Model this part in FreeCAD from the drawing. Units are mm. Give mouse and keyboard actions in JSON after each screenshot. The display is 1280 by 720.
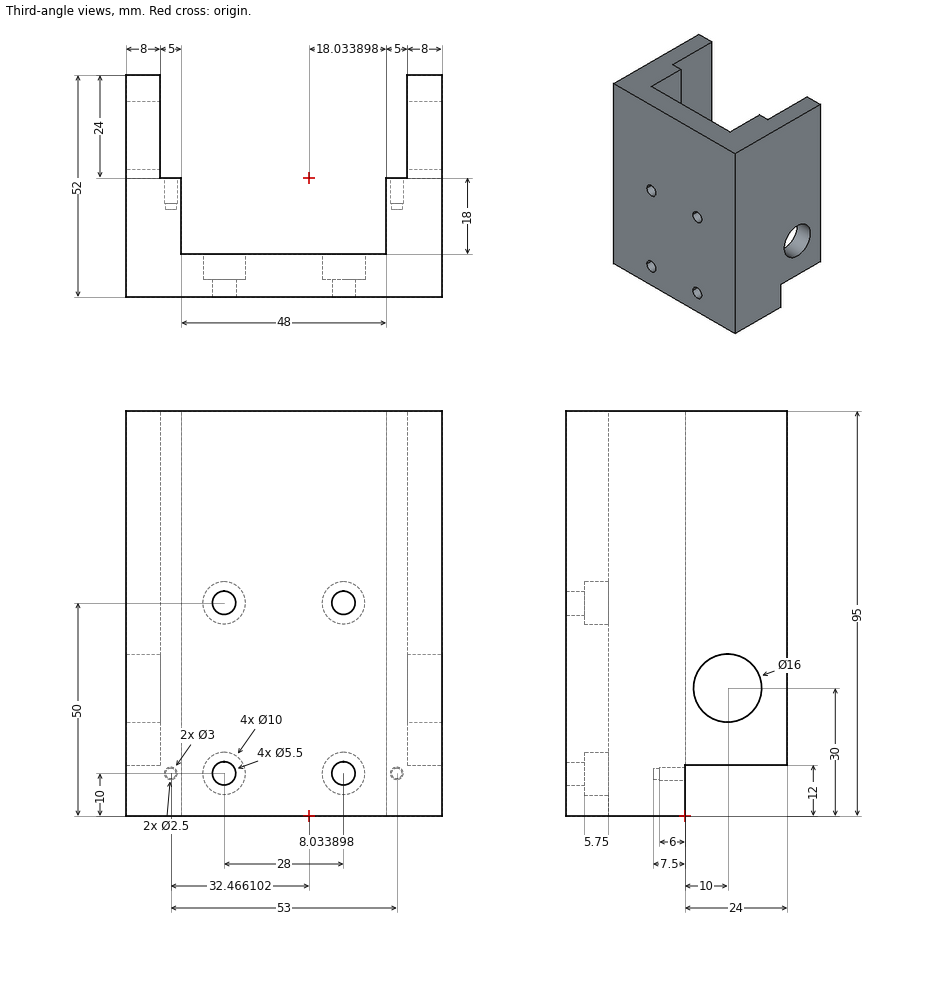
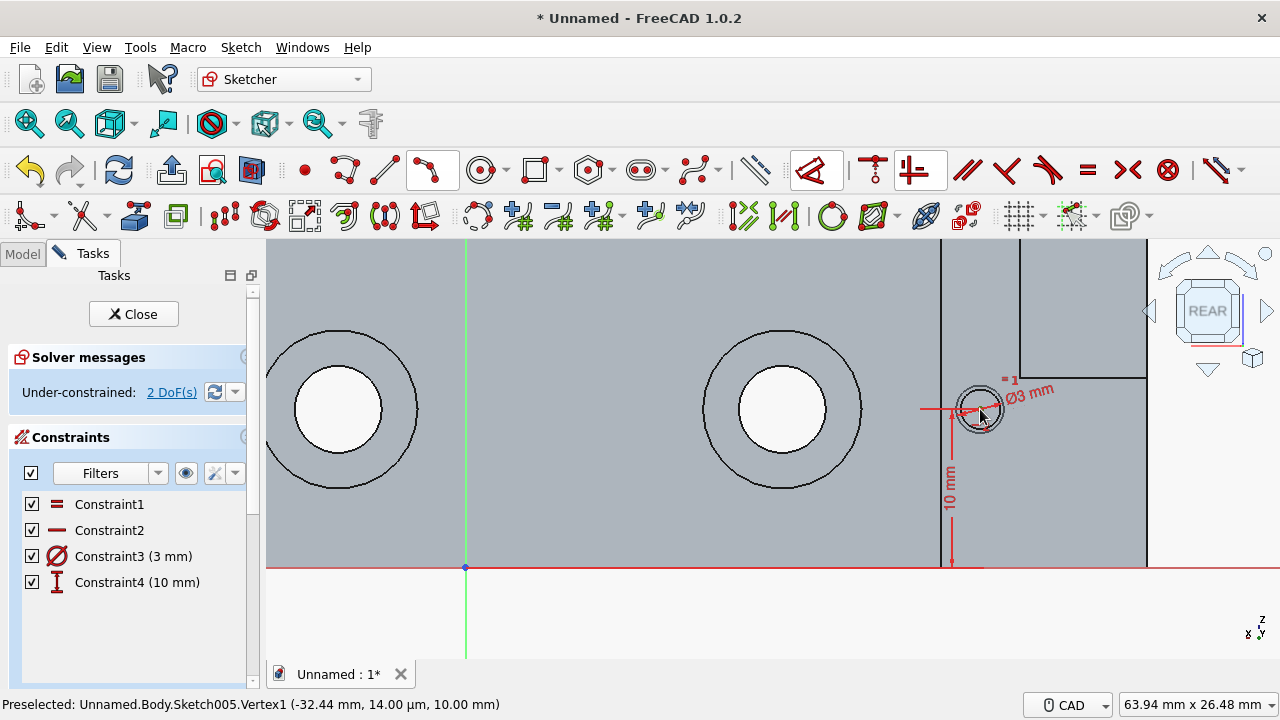
{"action": "scroll", "coordinate": [998, 393], "scroll_direction": "down", "scroll_amount": 2}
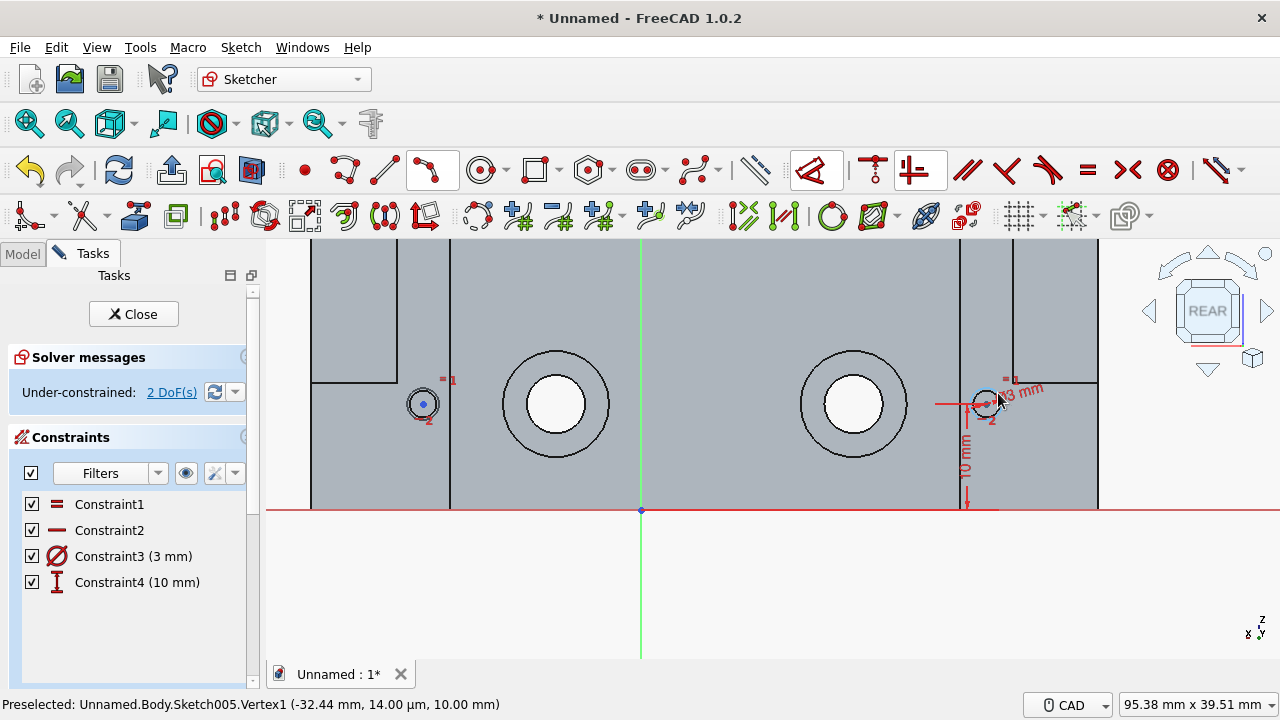
{"action": "left_click", "coordinate": [423, 404]}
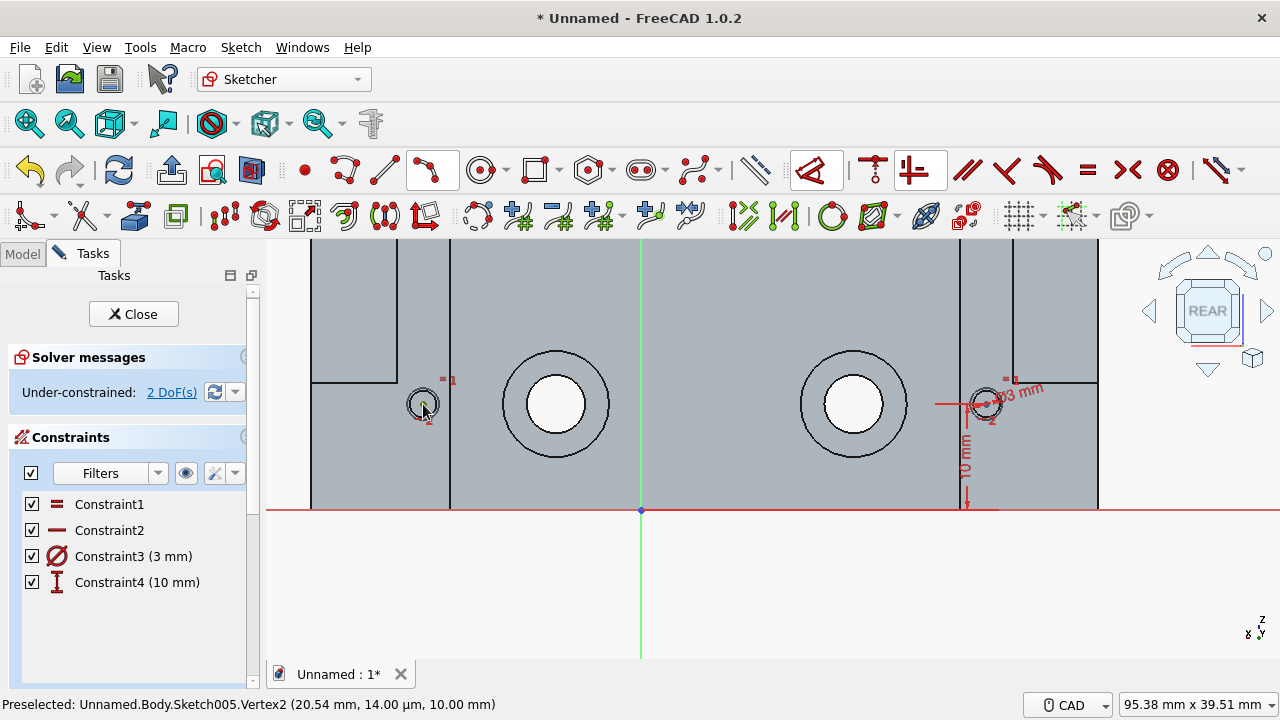
{"action": "key", "text": "l"}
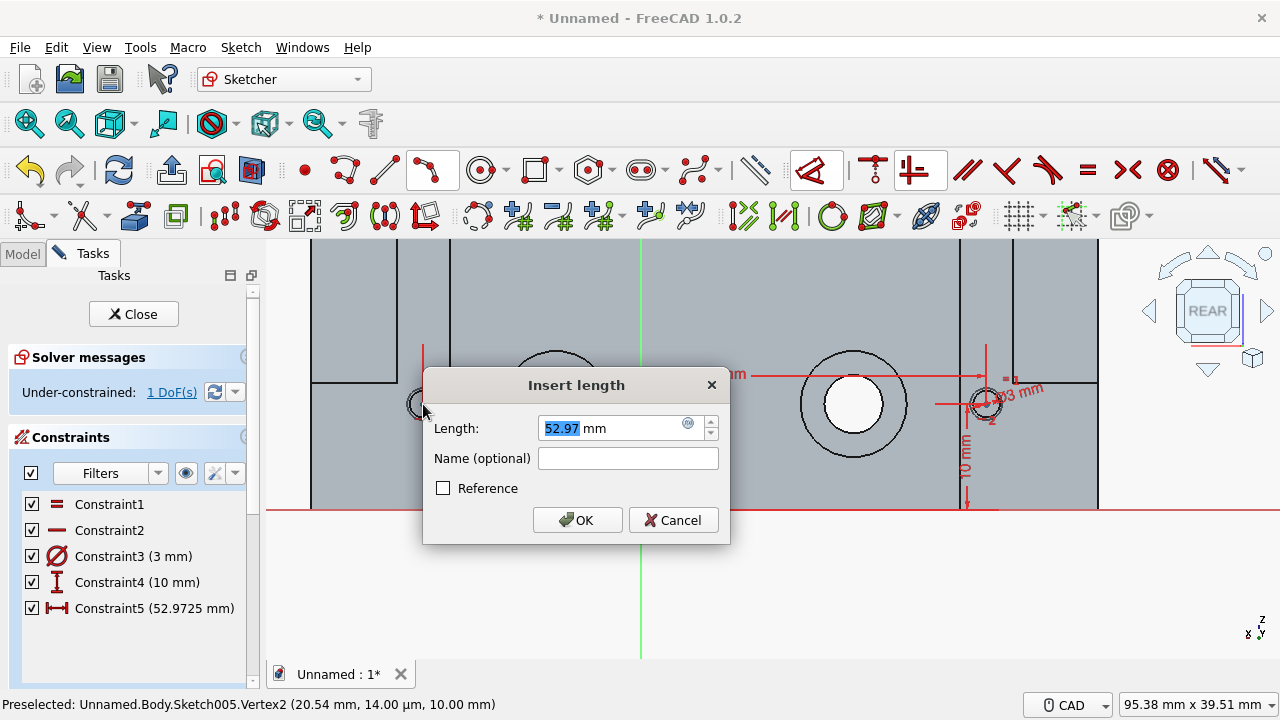
{"action": "type", "text": "53"}
{"action": "key", "text": "Return"}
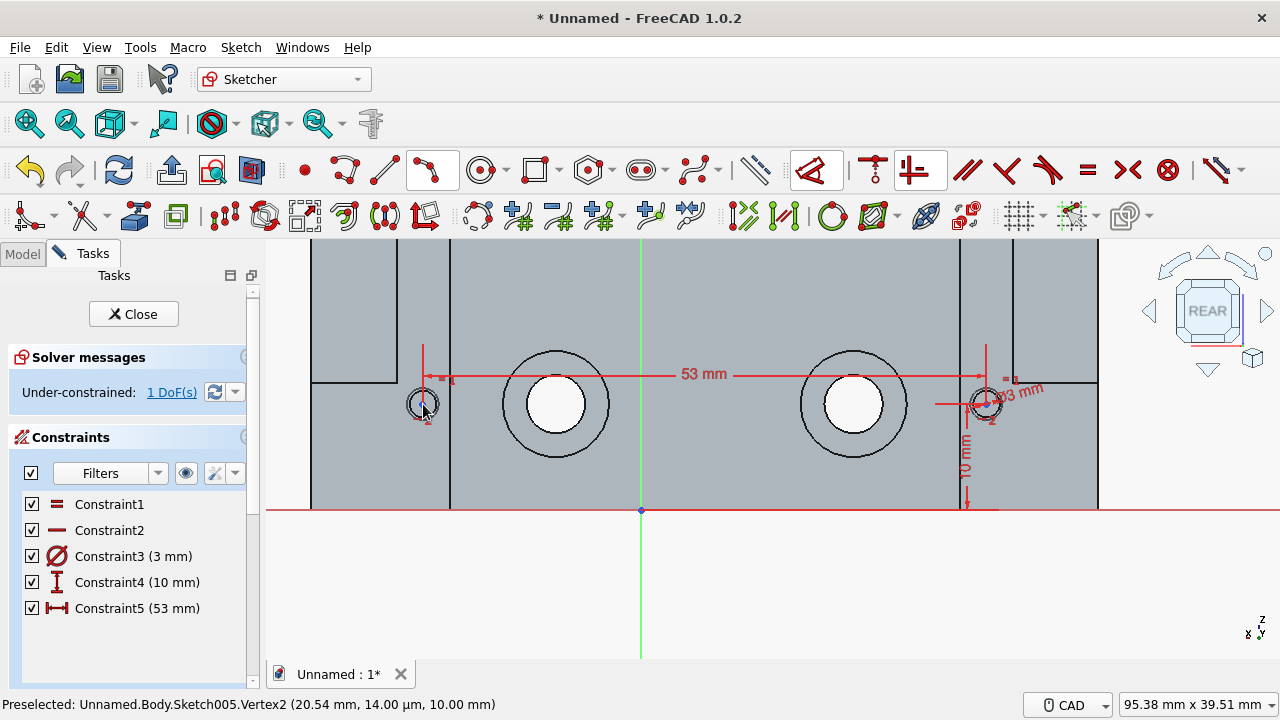
{"action": "left_click", "coordinate": [986, 404]}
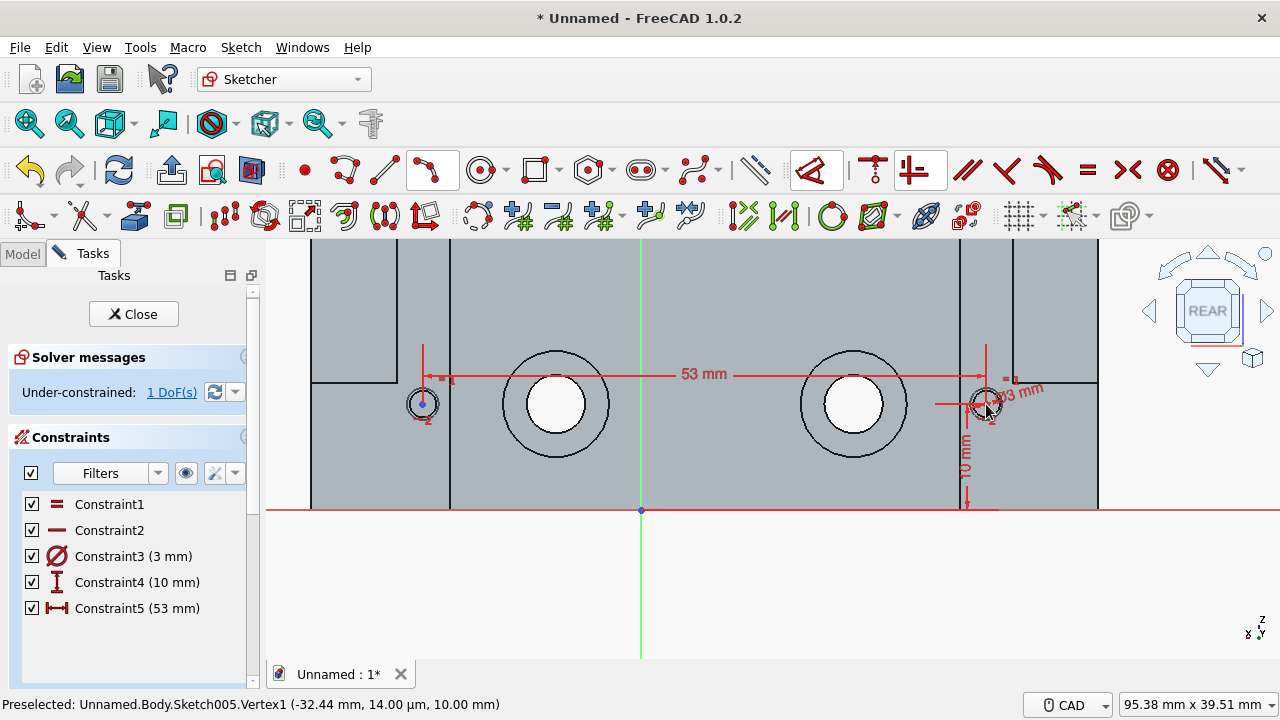
{"action": "key", "text": "l"}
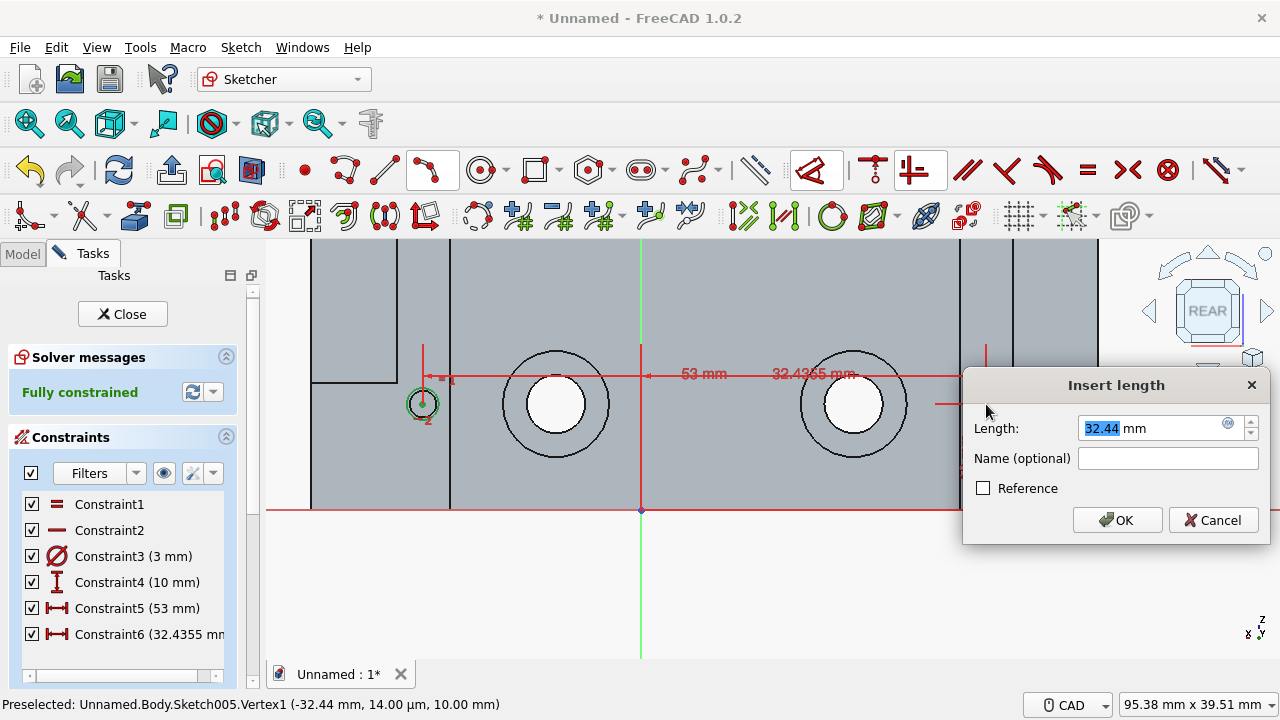
{"action": "type", "text": "32.466102"}
{"action": "key", "text": "Return"}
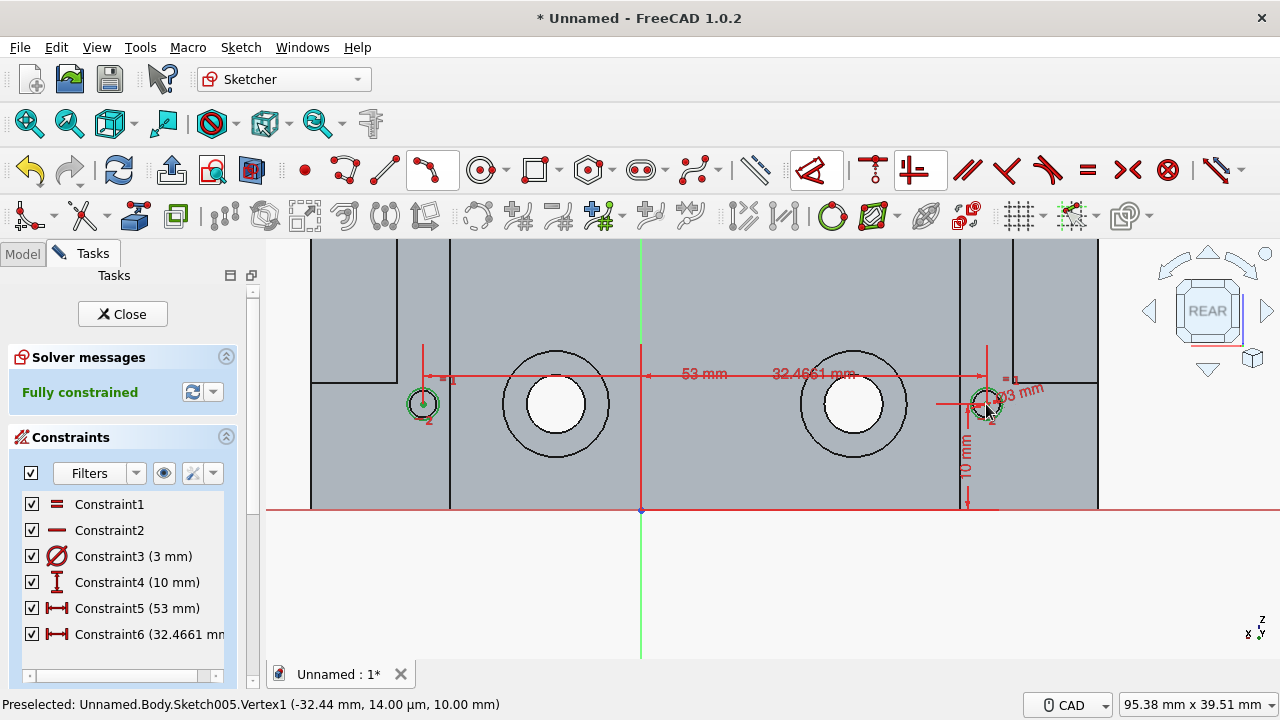
{"action": "left_click", "coordinate": [123, 314]}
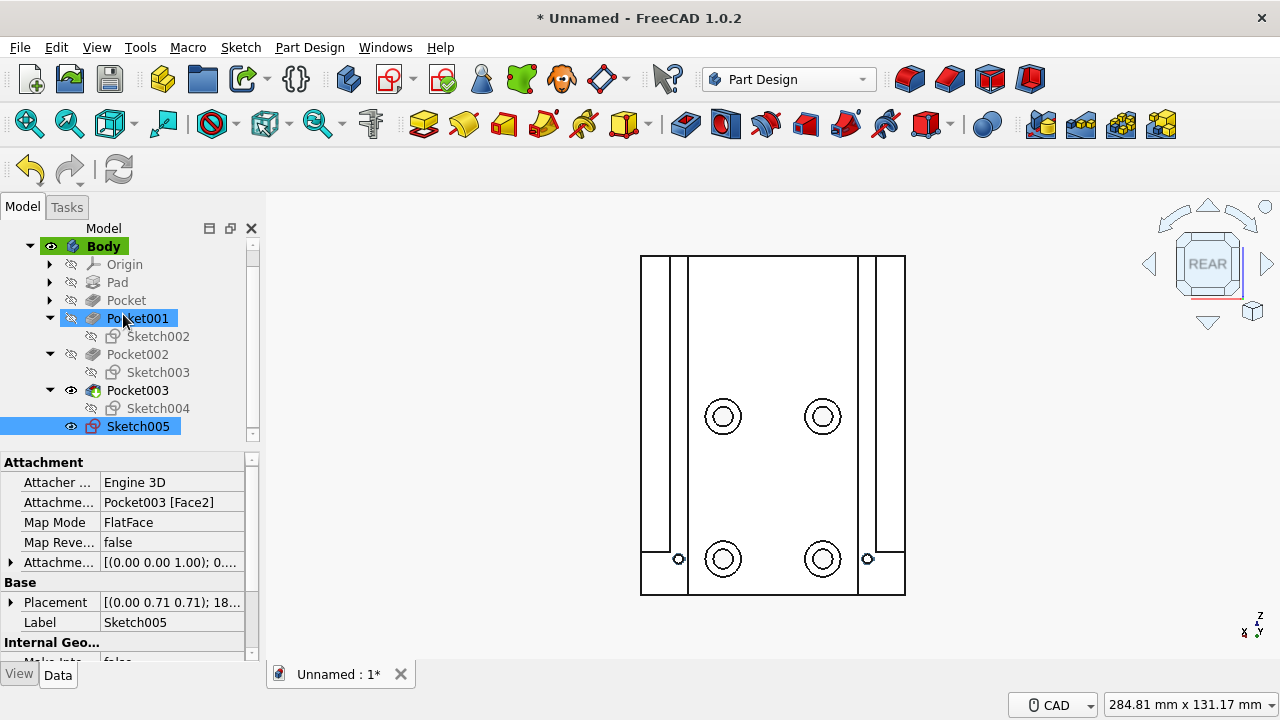
{"action": "left_click", "coordinate": [686, 124]}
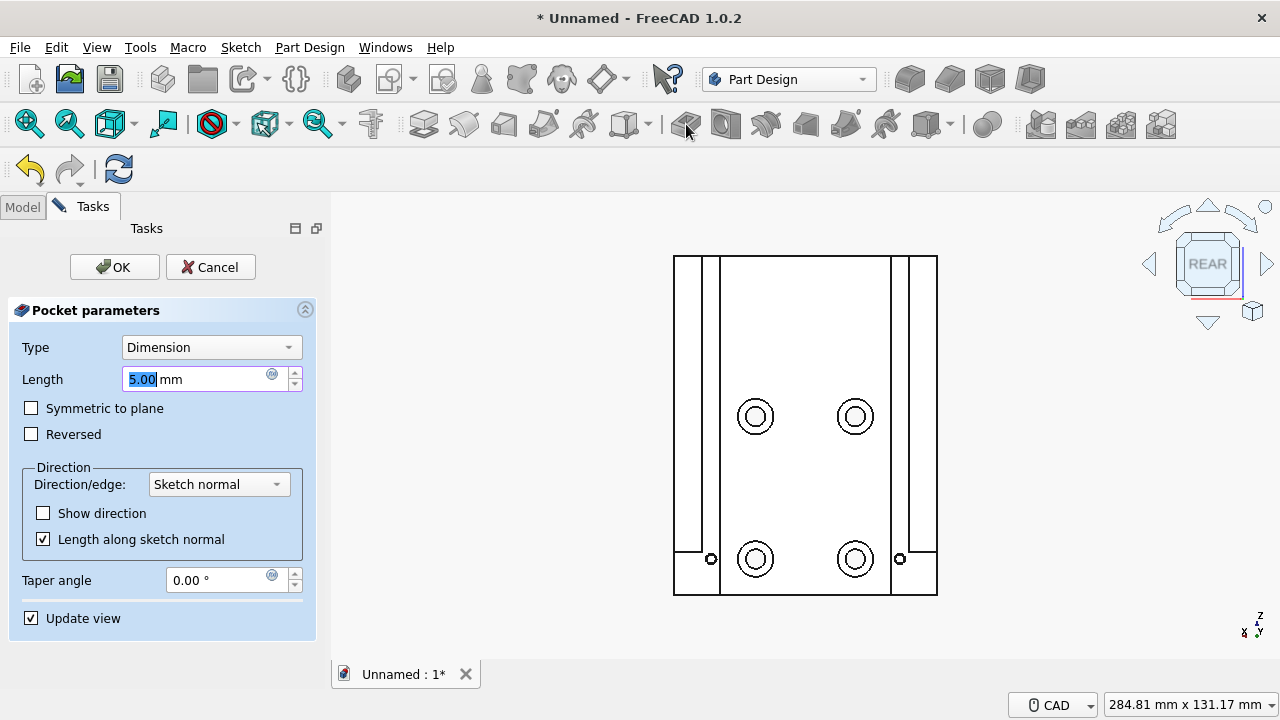
{"action": "type", "text": "6"}
{"action": "key", "text": "Tab"}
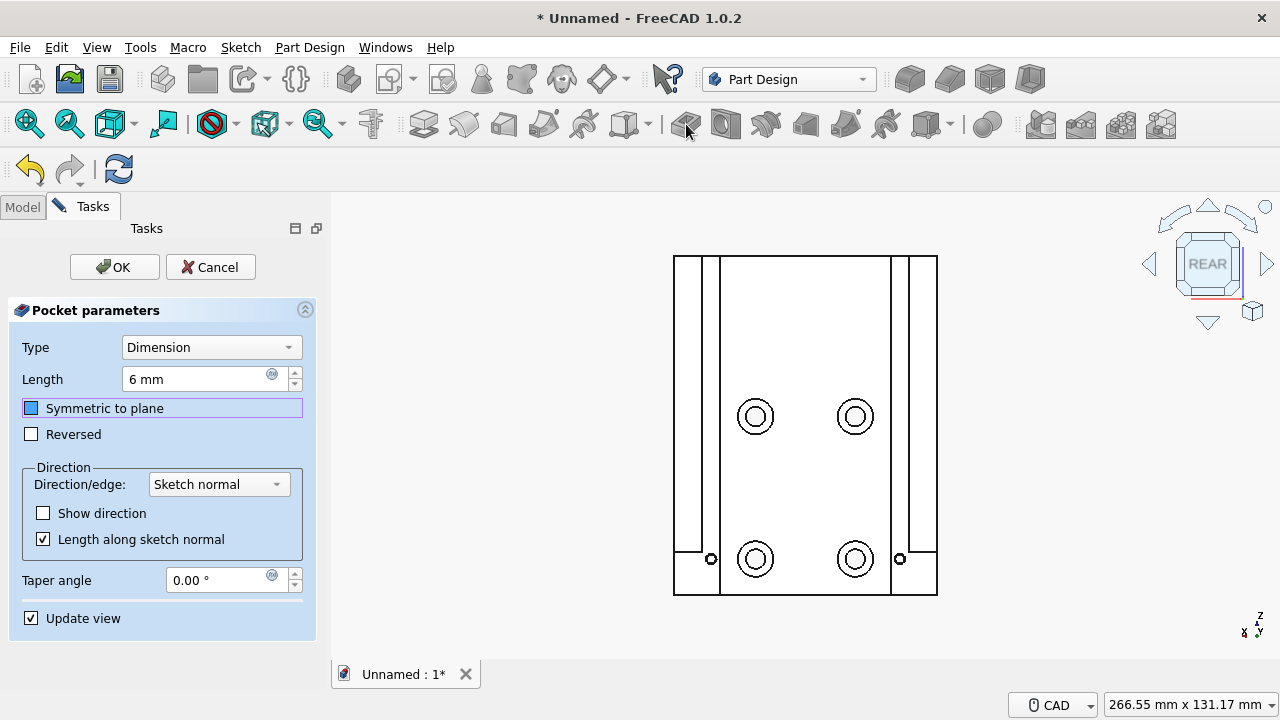
{"action": "left_click", "coordinate": [115, 267]}